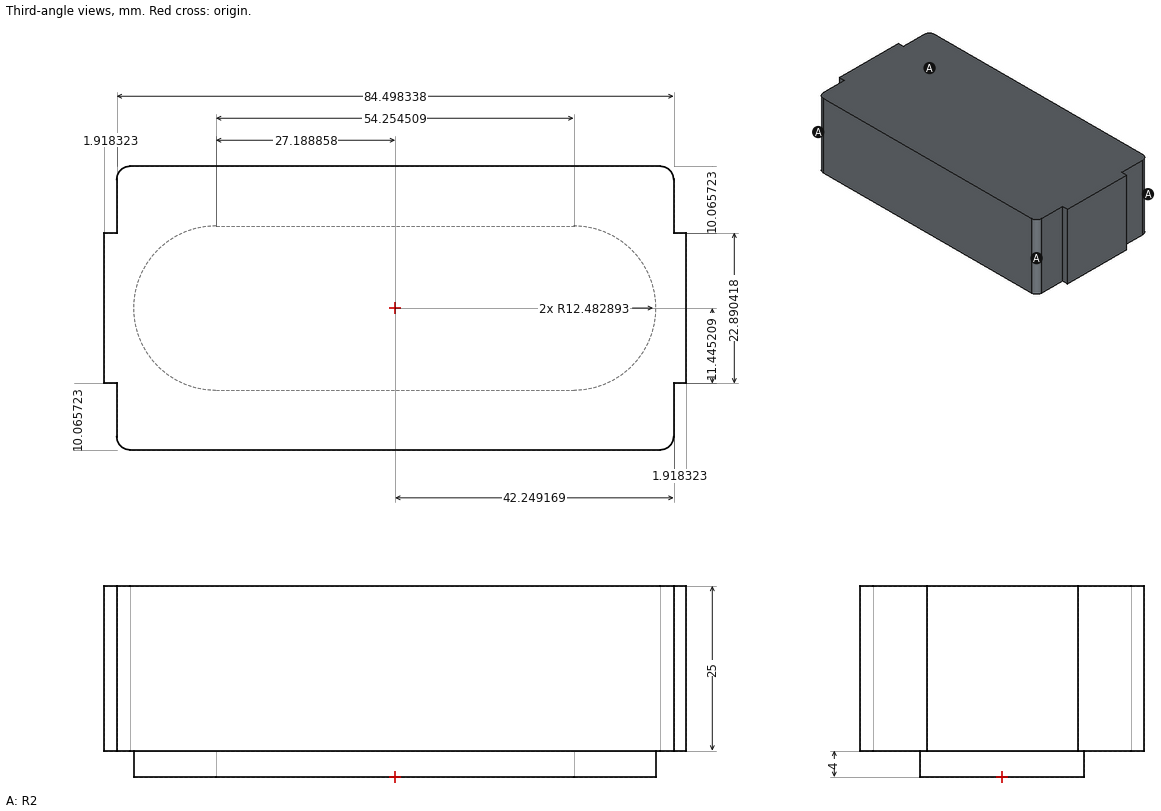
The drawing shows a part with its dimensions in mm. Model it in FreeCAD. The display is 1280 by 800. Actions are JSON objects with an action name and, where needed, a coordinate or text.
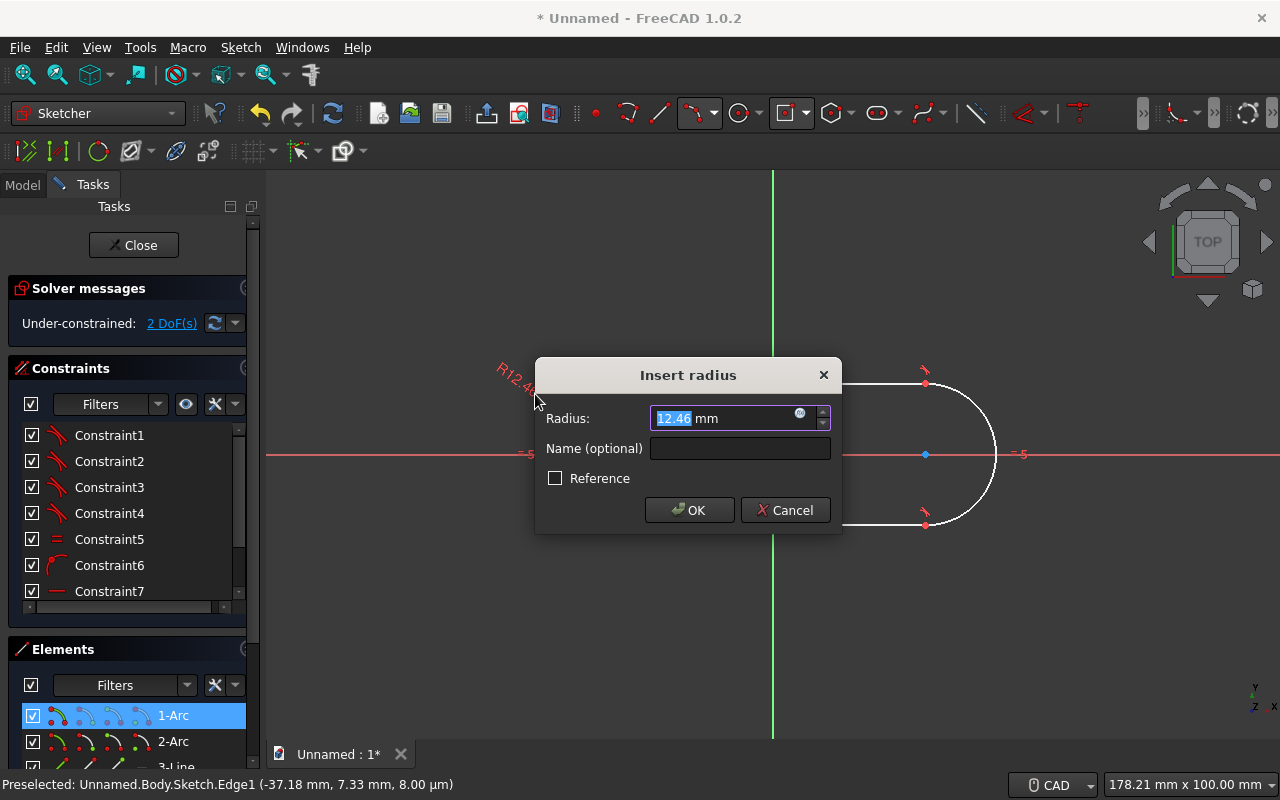
{"action": "type", "text": "12.482893"}
{"action": "key", "text": "Return"}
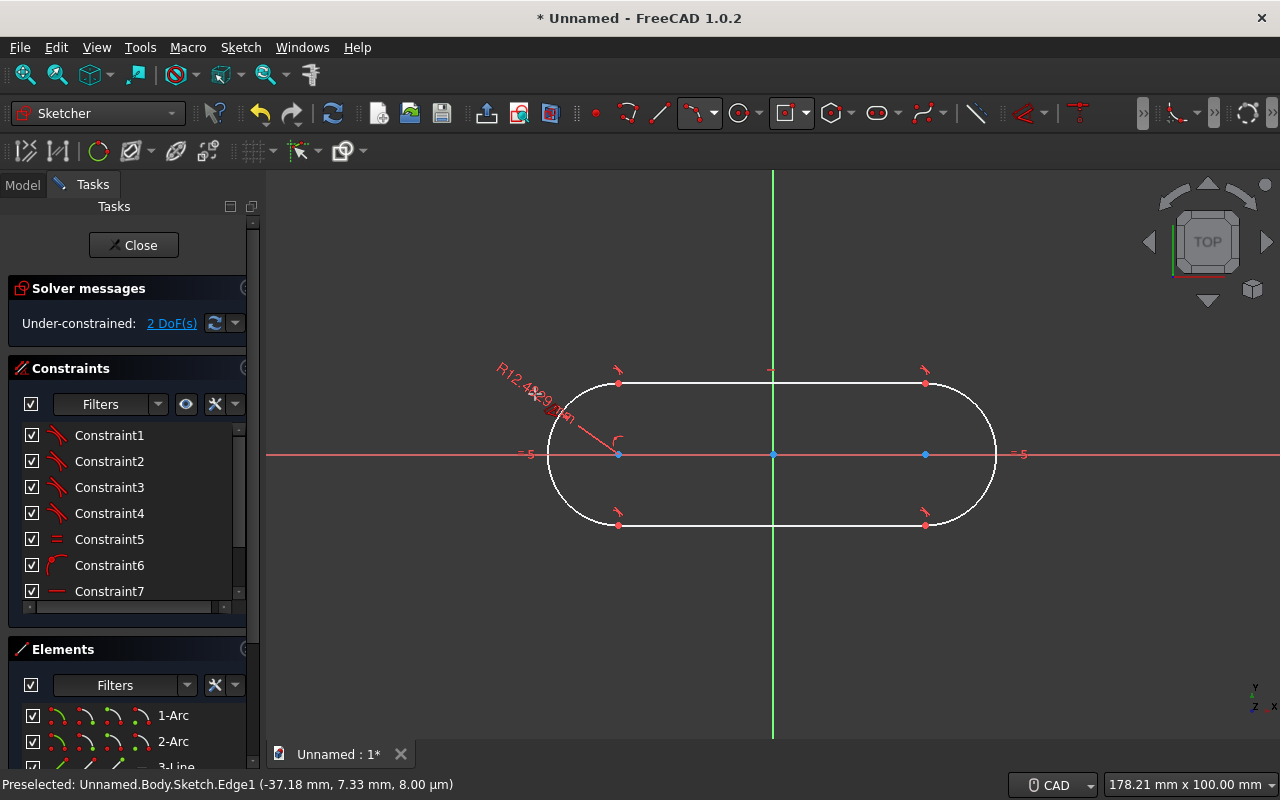
{"action": "left_click", "coordinate": [711, 383]}
{"action": "left_click", "coordinate": [702, 349]}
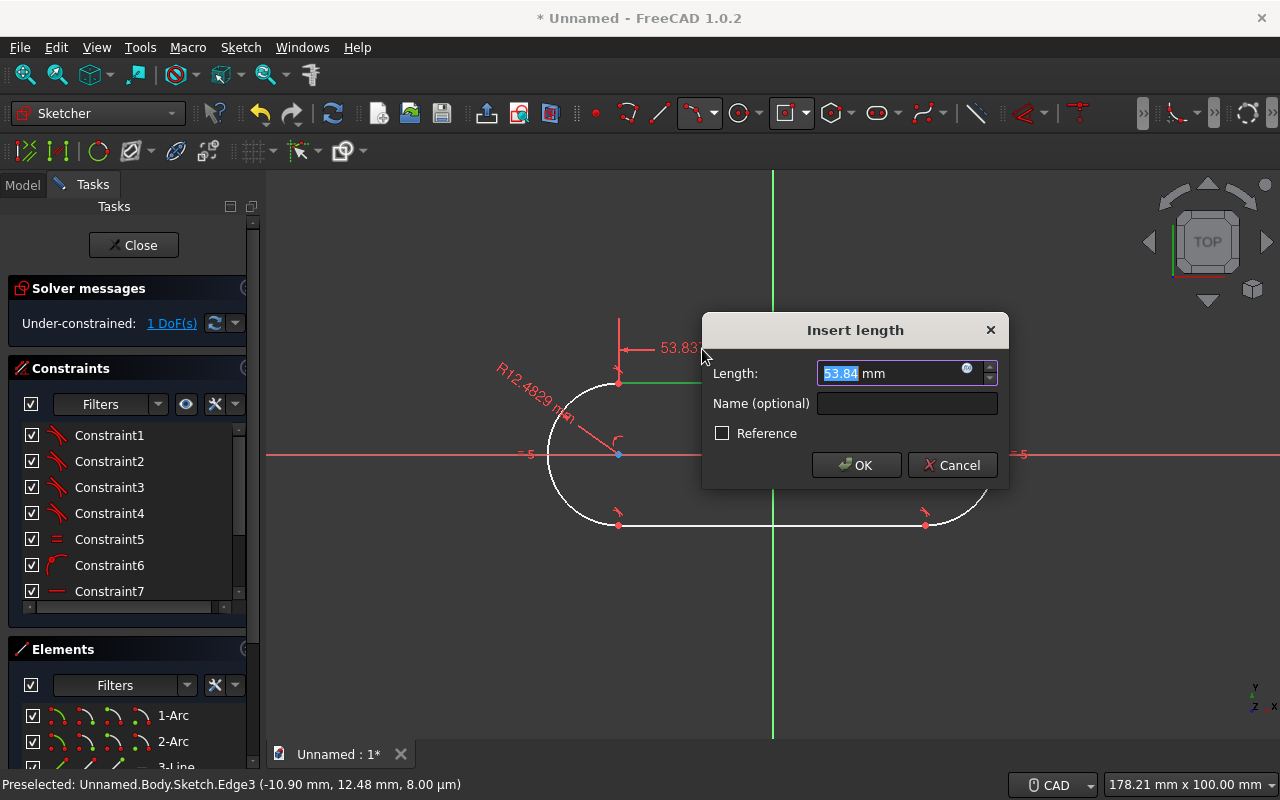
{"action": "type", "text": "54.254509"}
{"action": "key", "text": "Return"}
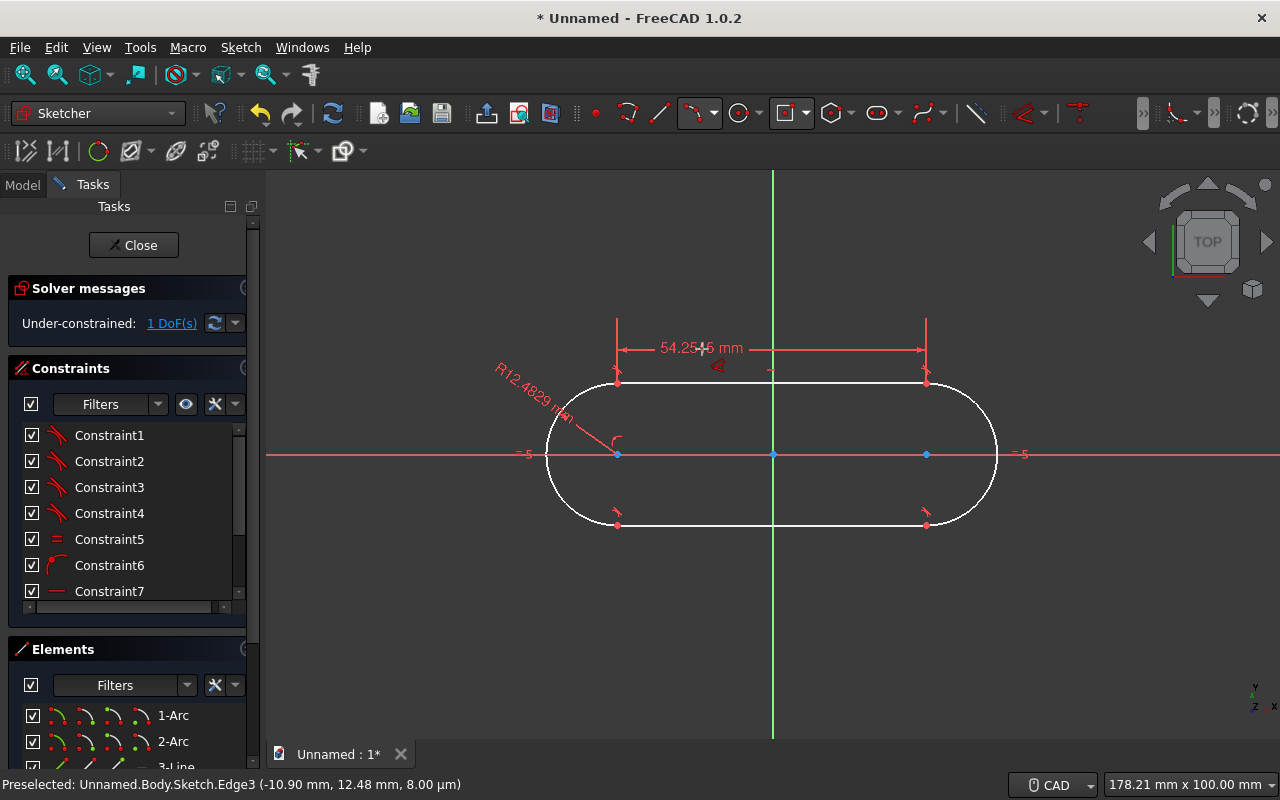
{"action": "left_click", "coordinate": [617, 383]}
{"action": "left_click", "coordinate": [695, 488]}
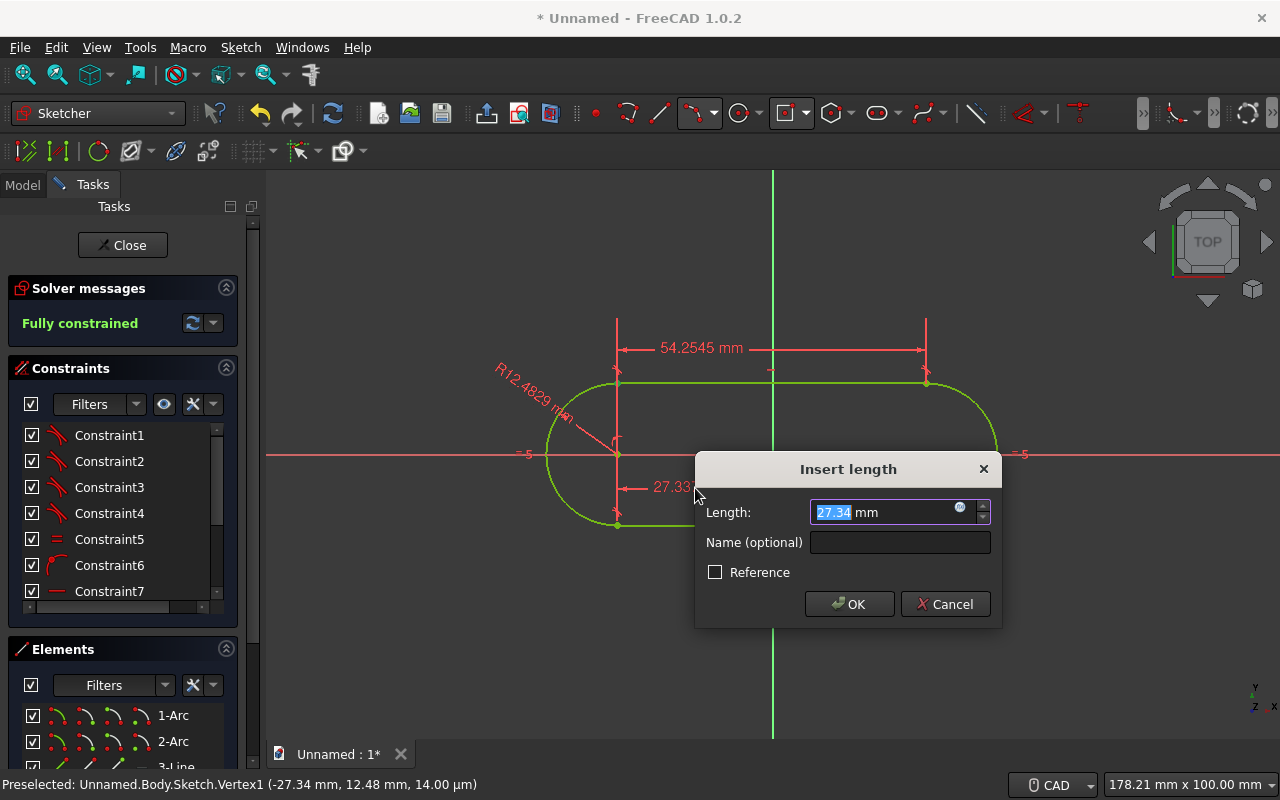
{"action": "type", "text": "27.188858"}
{"action": "key", "text": "Return"}
{"action": "key", "text": "Escape"}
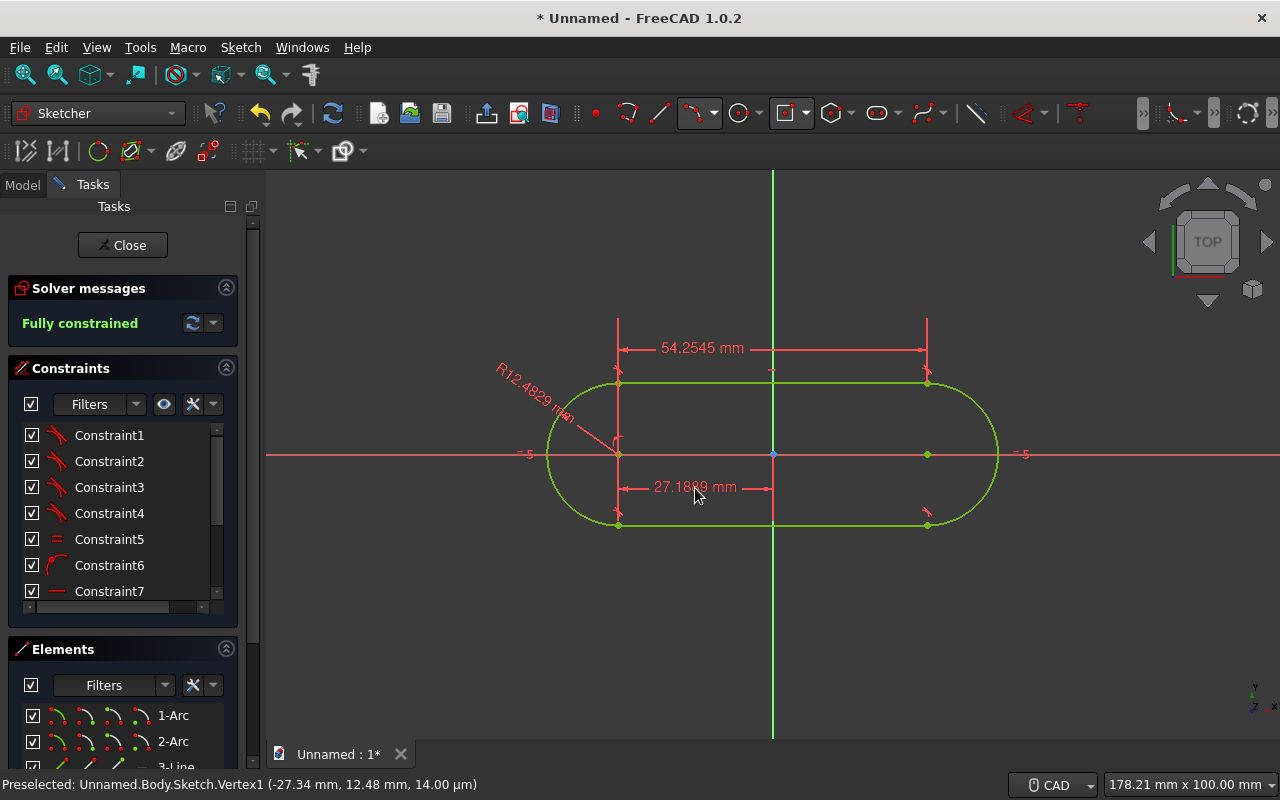
{"action": "left_click", "coordinate": [123, 245]}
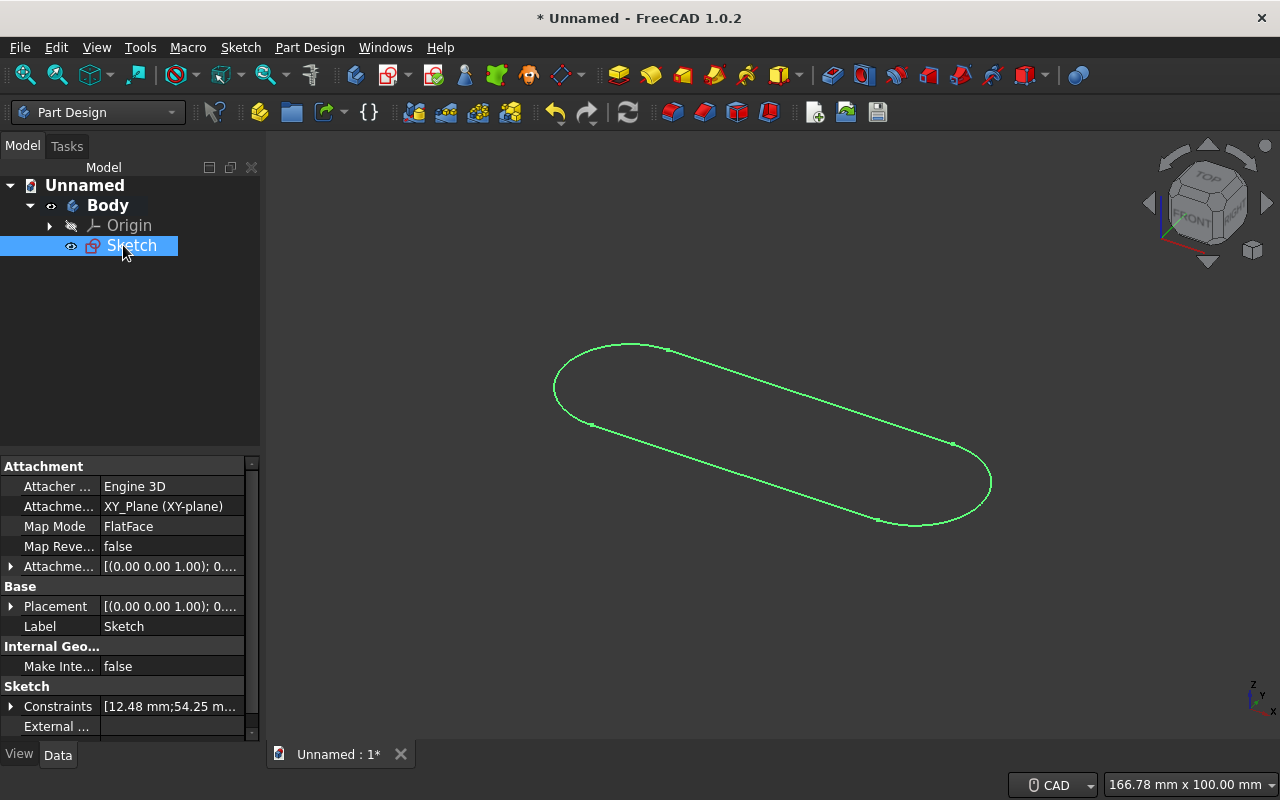
{"action": "left_click", "coordinate": [620, 76]}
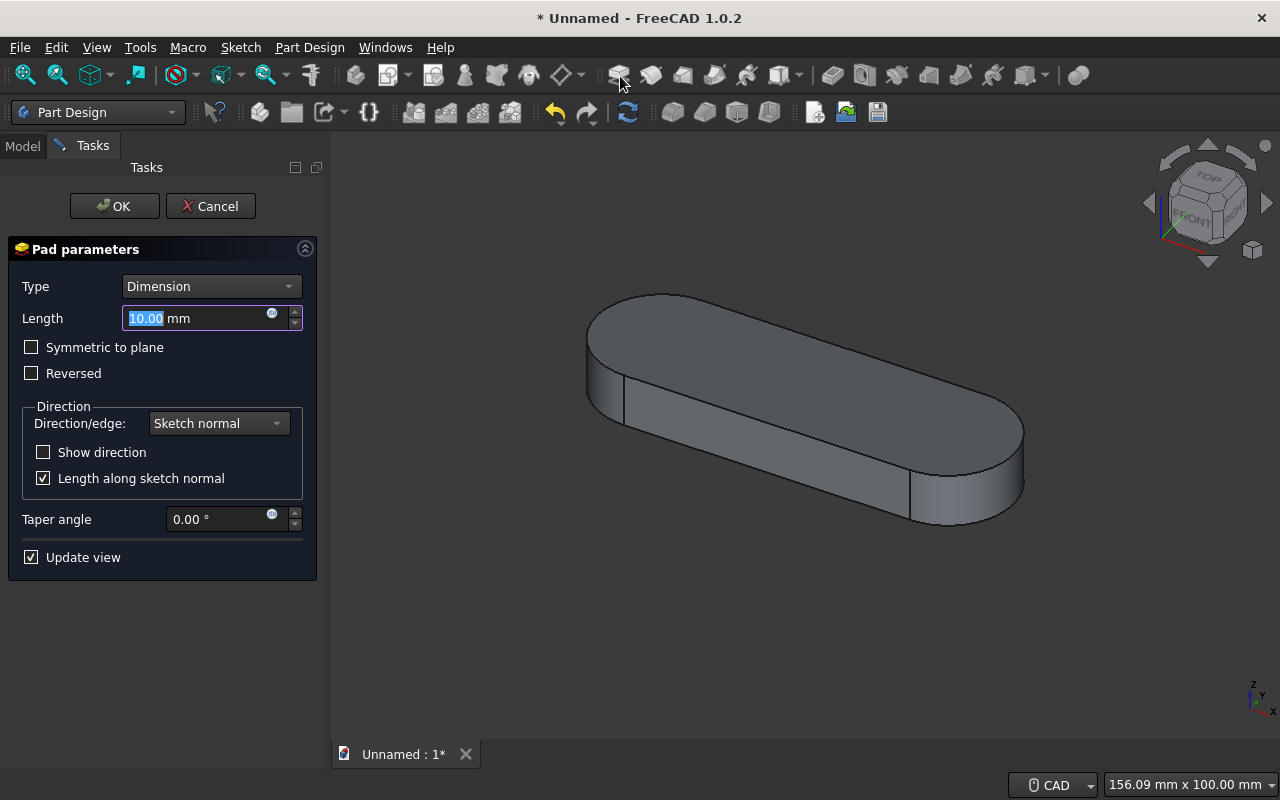
{"action": "type", "text": "4"}
{"action": "key", "text": "Tab"}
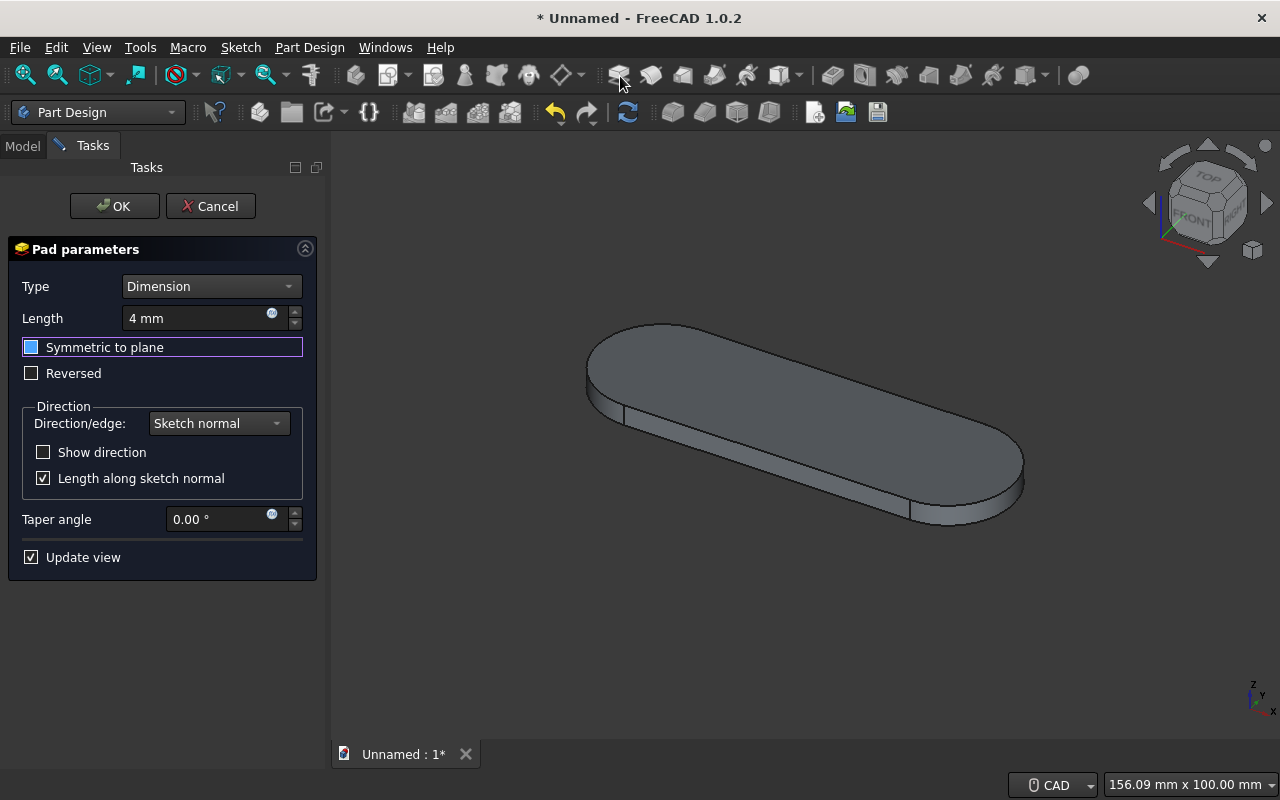
{"action": "left_click", "coordinate": [115, 206]}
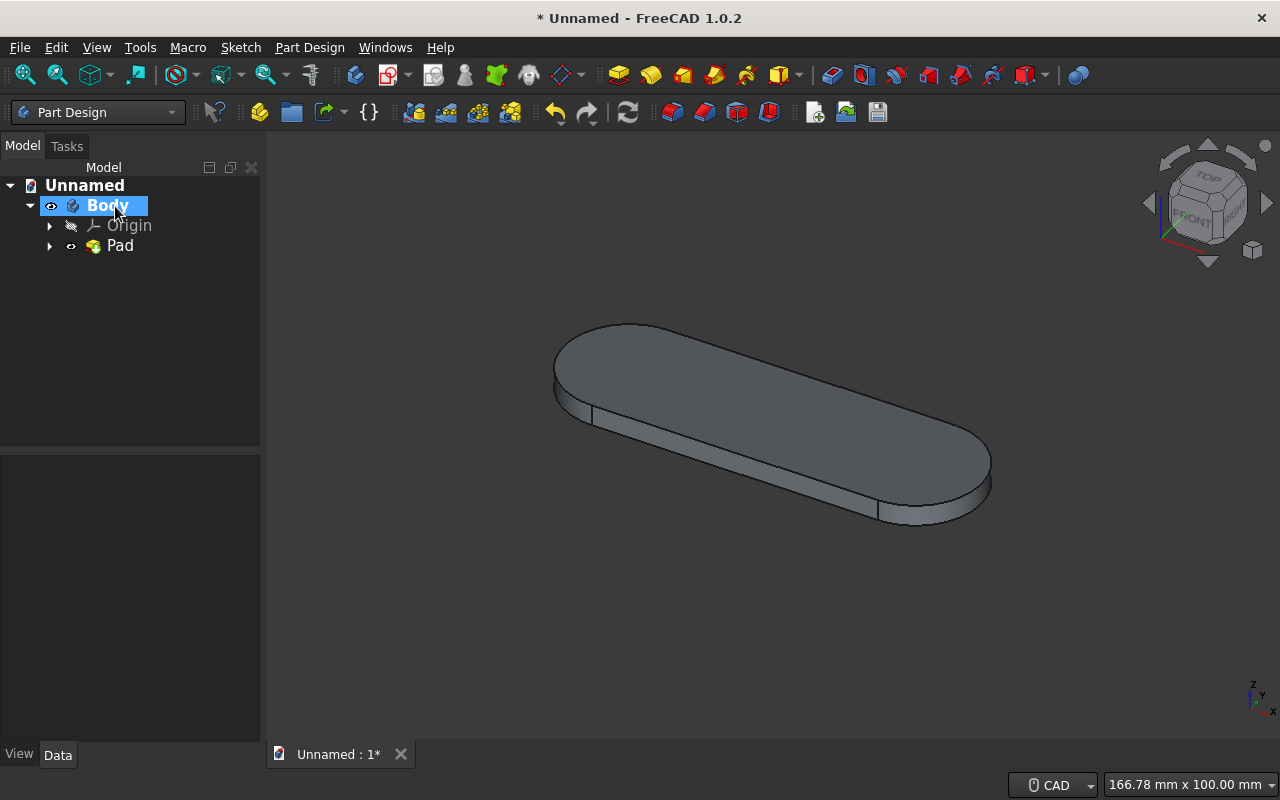
{"action": "left_click", "coordinate": [773, 414]}